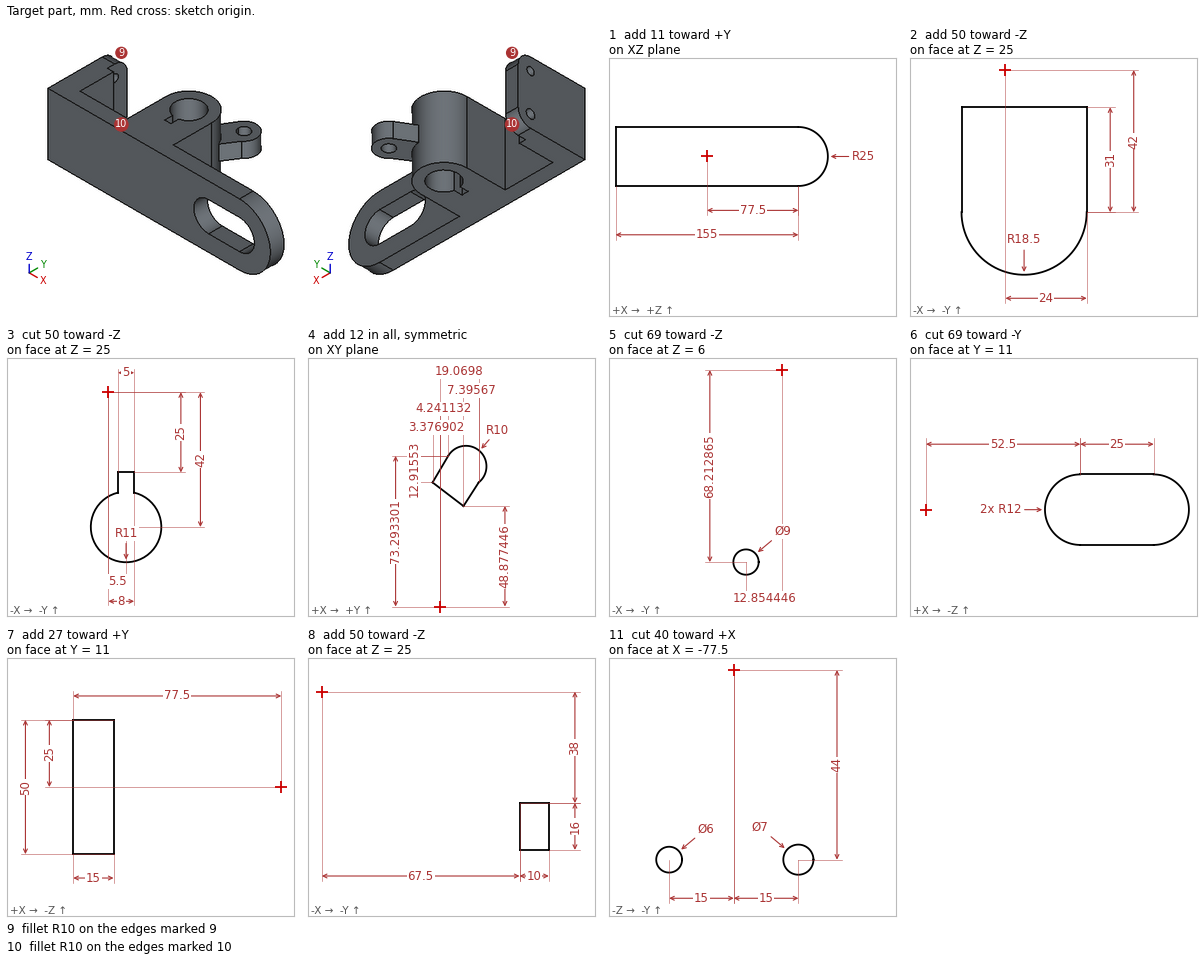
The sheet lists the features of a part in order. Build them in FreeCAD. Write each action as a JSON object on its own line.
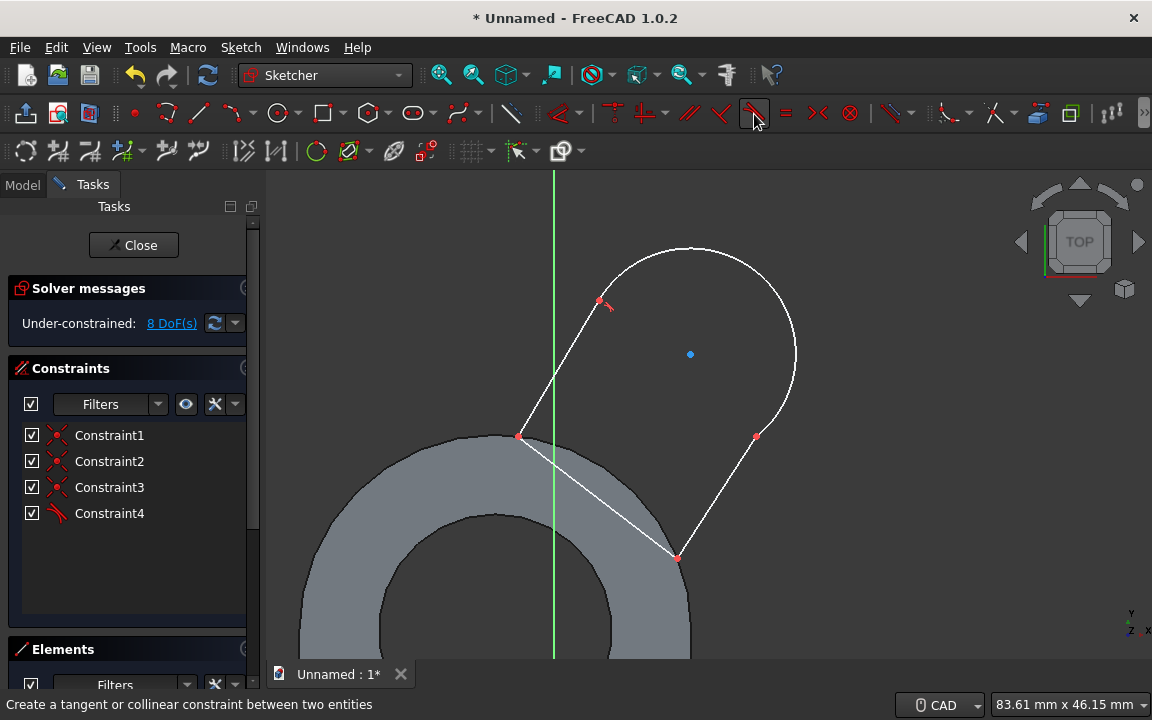
{"action": "left_click", "coordinate": [558, 114]}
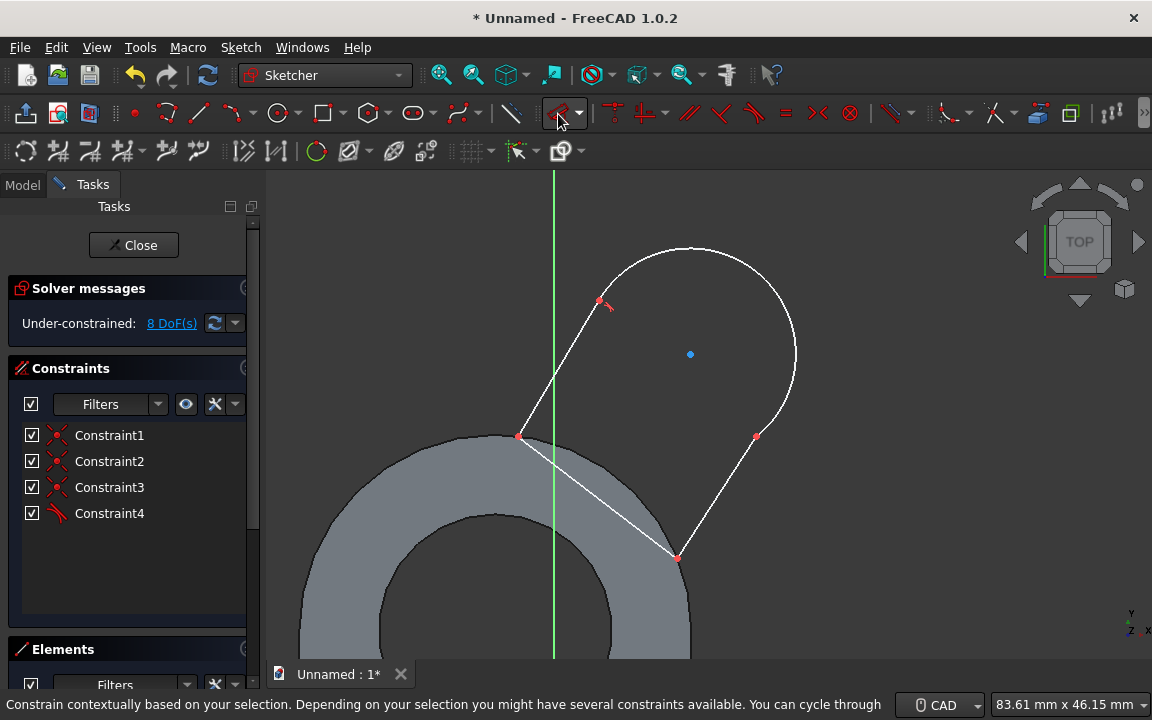
{"action": "left_click", "coordinate": [795, 338]}
{"action": "left_click", "coordinate": [827, 333]}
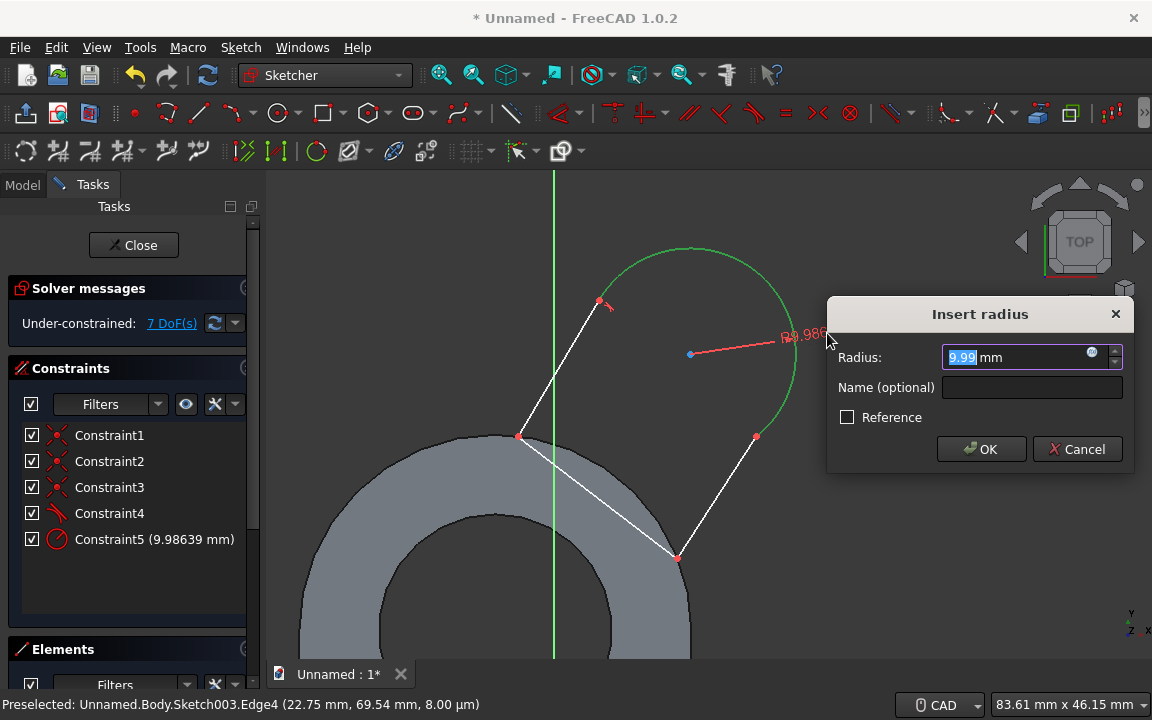
{"action": "type", "text": "10"}
{"action": "key", "text": "Return"}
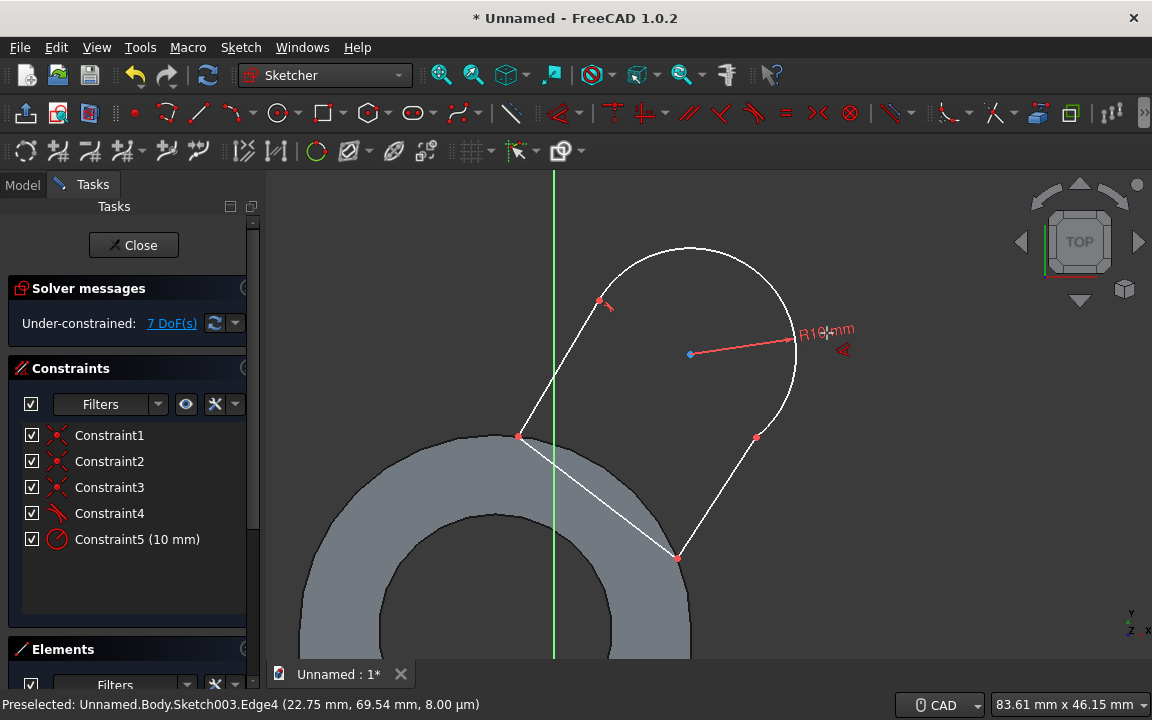
{"action": "left_click", "coordinate": [756, 437]}
{"action": "left_click", "coordinate": [655, 403]}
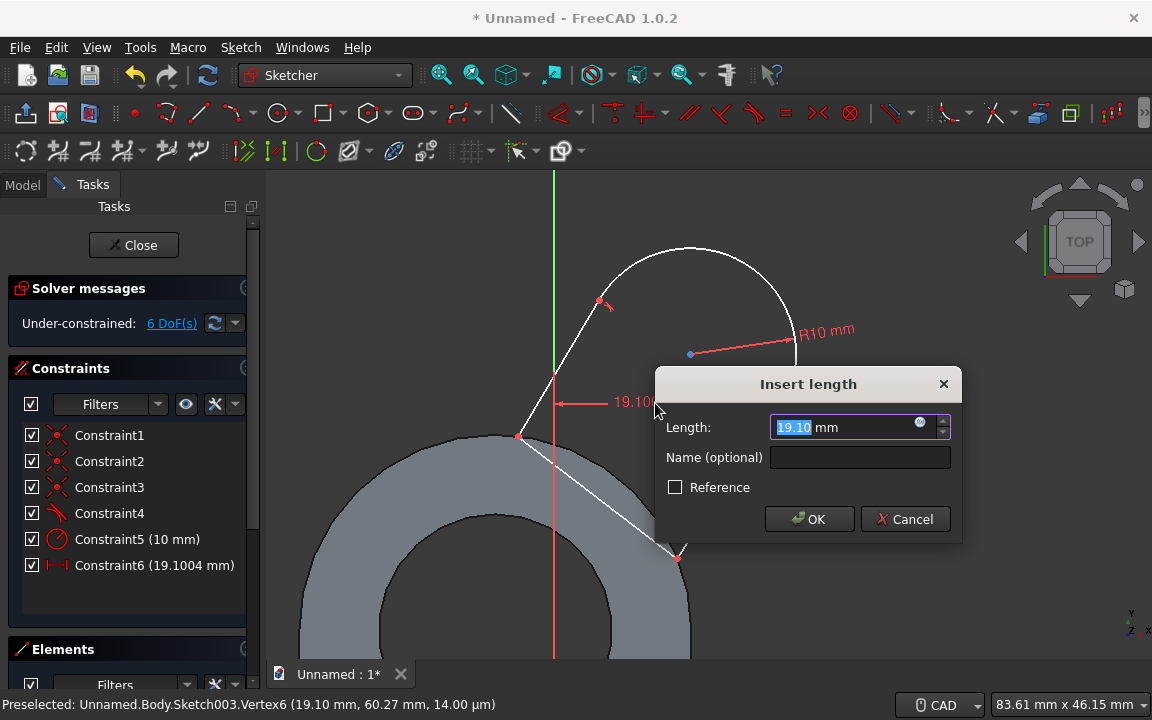
{"action": "type", "text": "19.0698"}
{"action": "key", "text": "Return"}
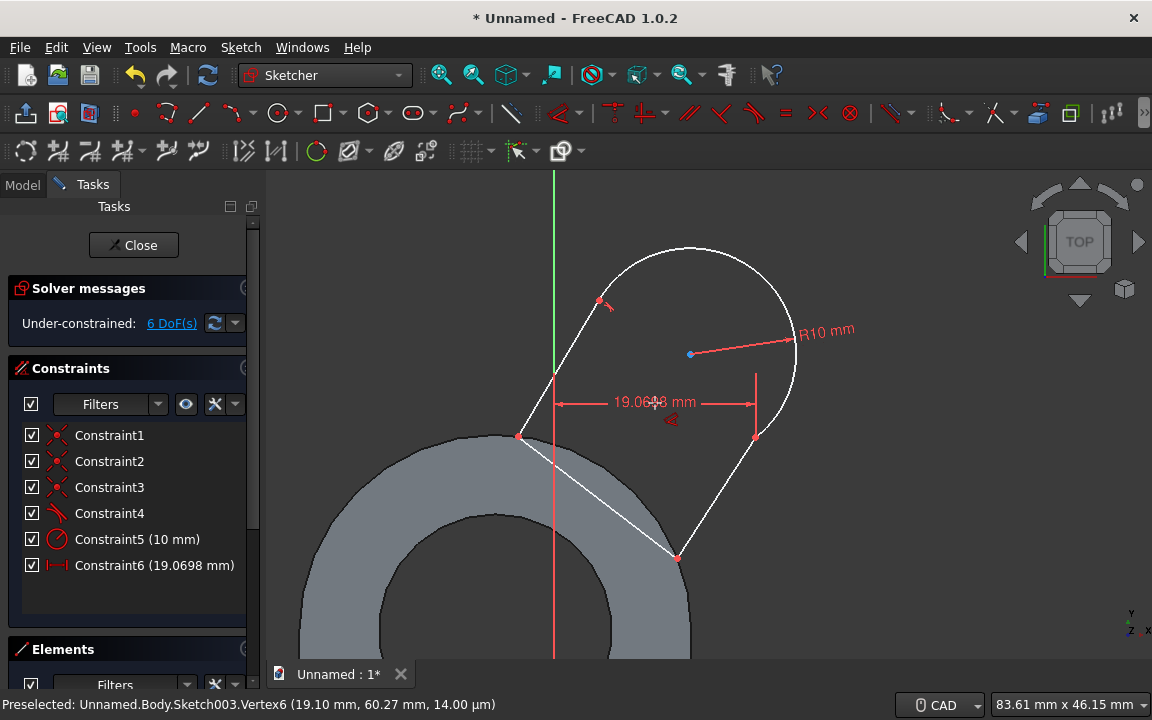
{"action": "left_click", "coordinate": [701, 523]}
{"action": "left_click", "coordinate": [716, 593]}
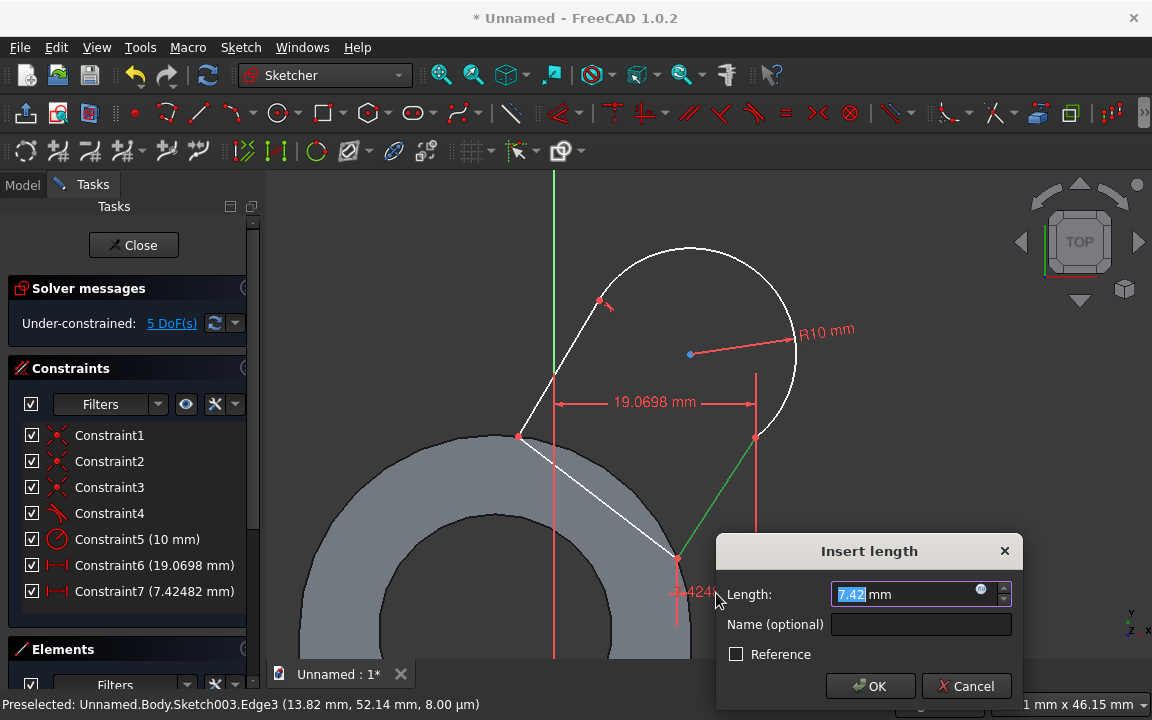
{"action": "type", "text": "7.39567"}
{"action": "key", "text": "Return"}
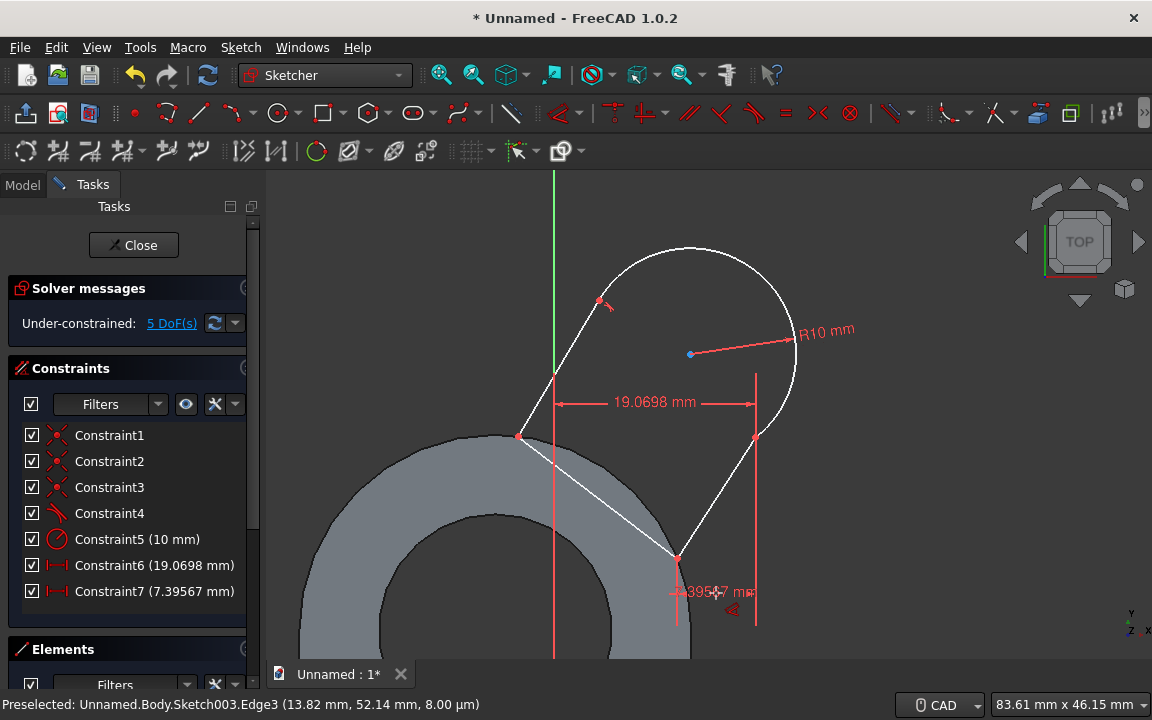
{"action": "left_click", "coordinate": [599, 300]}
{"action": "left_click", "coordinate": [576, 266]}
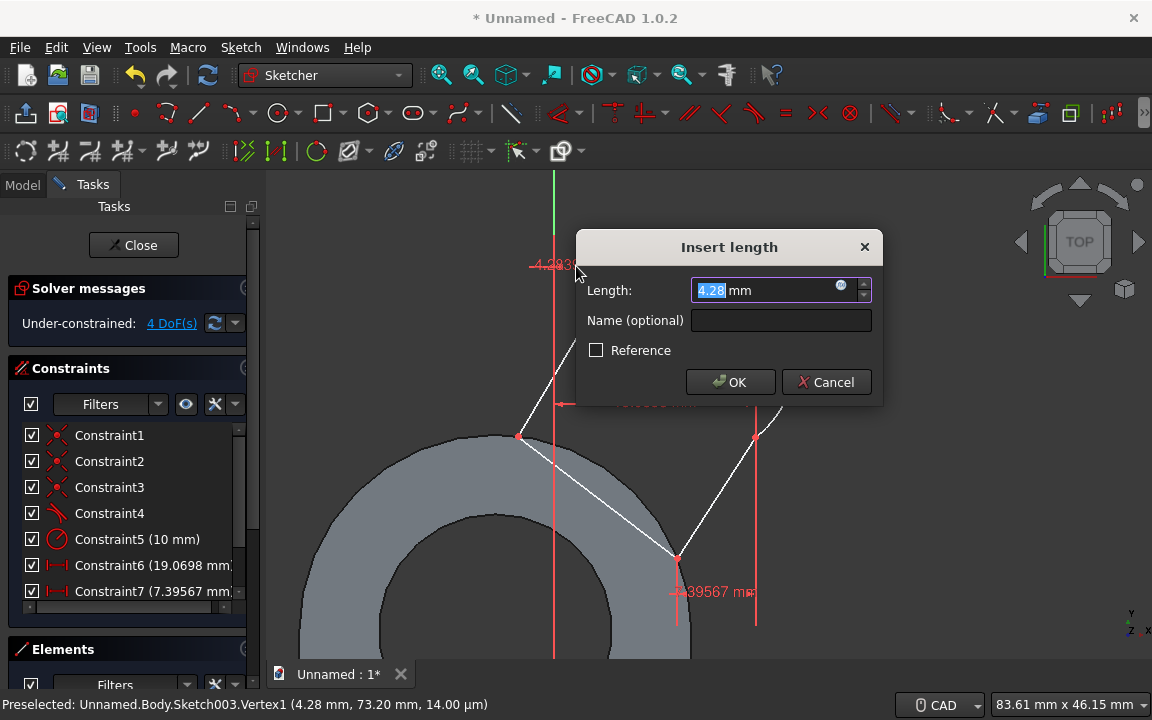
{"action": "type", "text": "4.241132"}
{"action": "key", "text": "Return"}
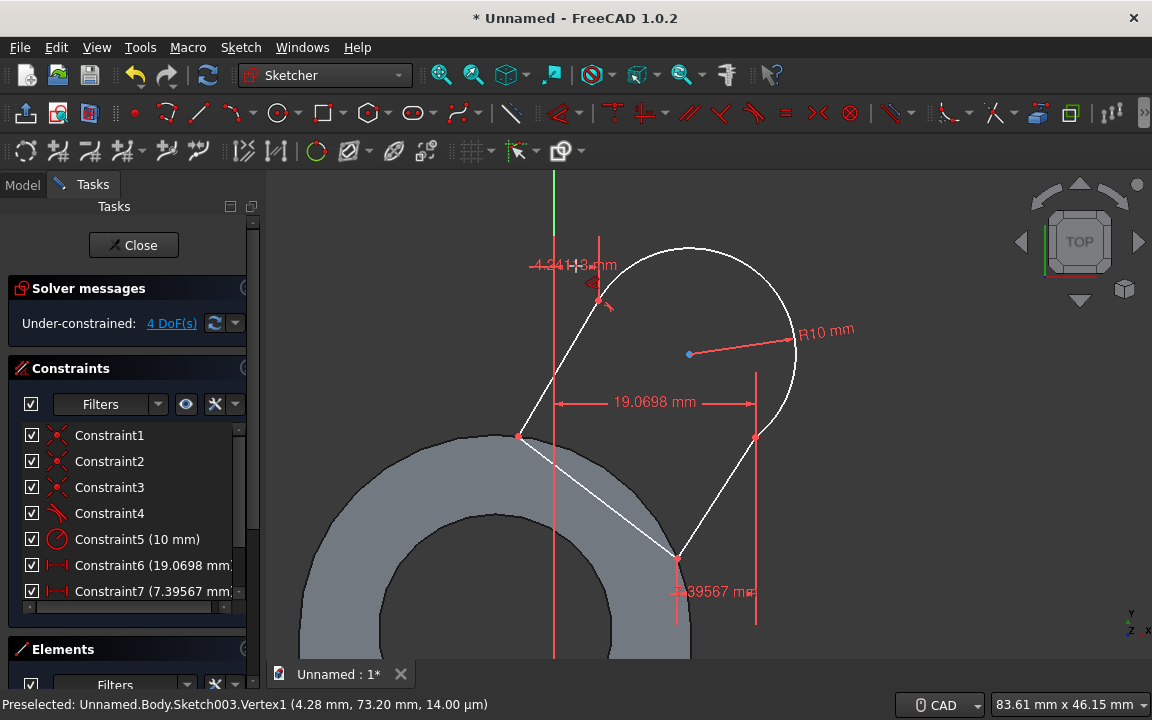
{"action": "left_click", "coordinate": [518, 437]}
{"action": "left_click", "coordinate": [536, 379]}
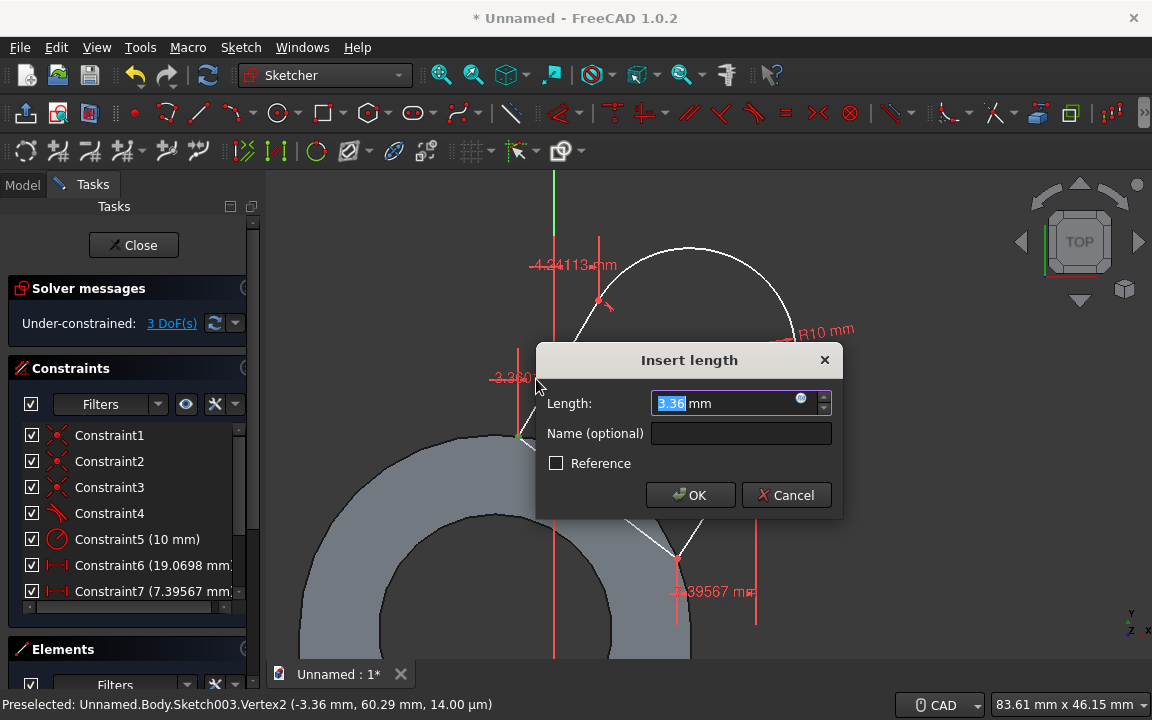
{"action": "type", "text": "3.376902"}
{"action": "key", "text": "Return"}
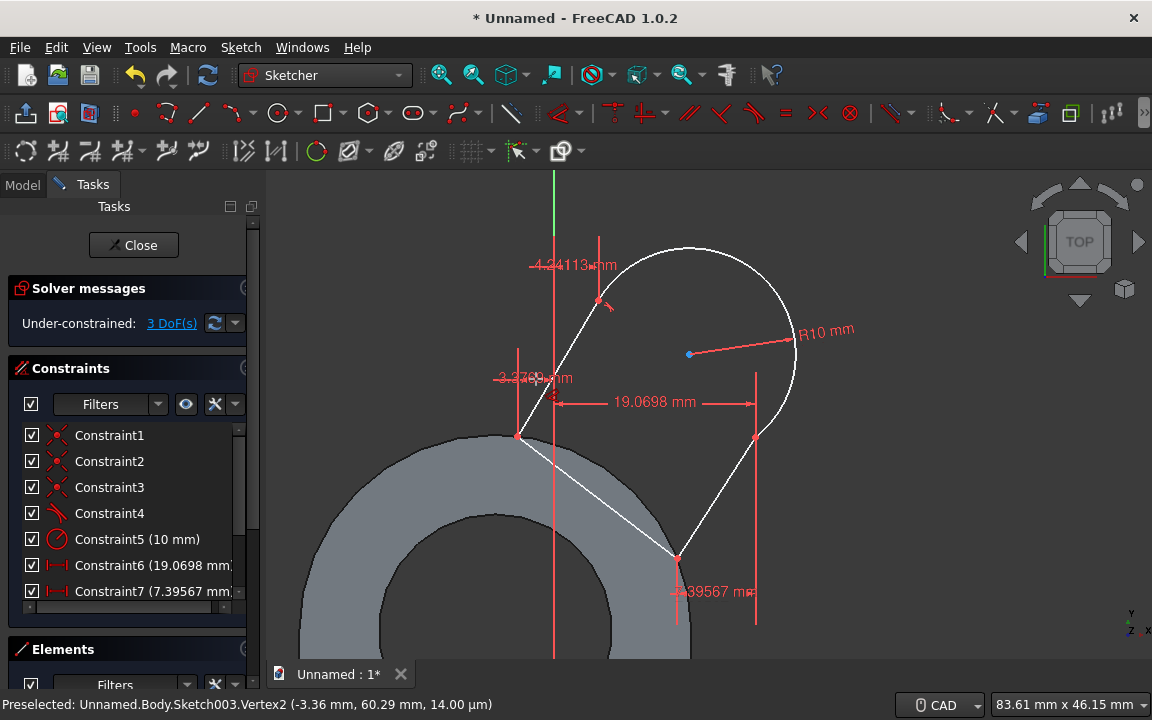
{"action": "left_click", "coordinate": [574, 341]}
{"action": "left_click", "coordinate": [484, 337]}